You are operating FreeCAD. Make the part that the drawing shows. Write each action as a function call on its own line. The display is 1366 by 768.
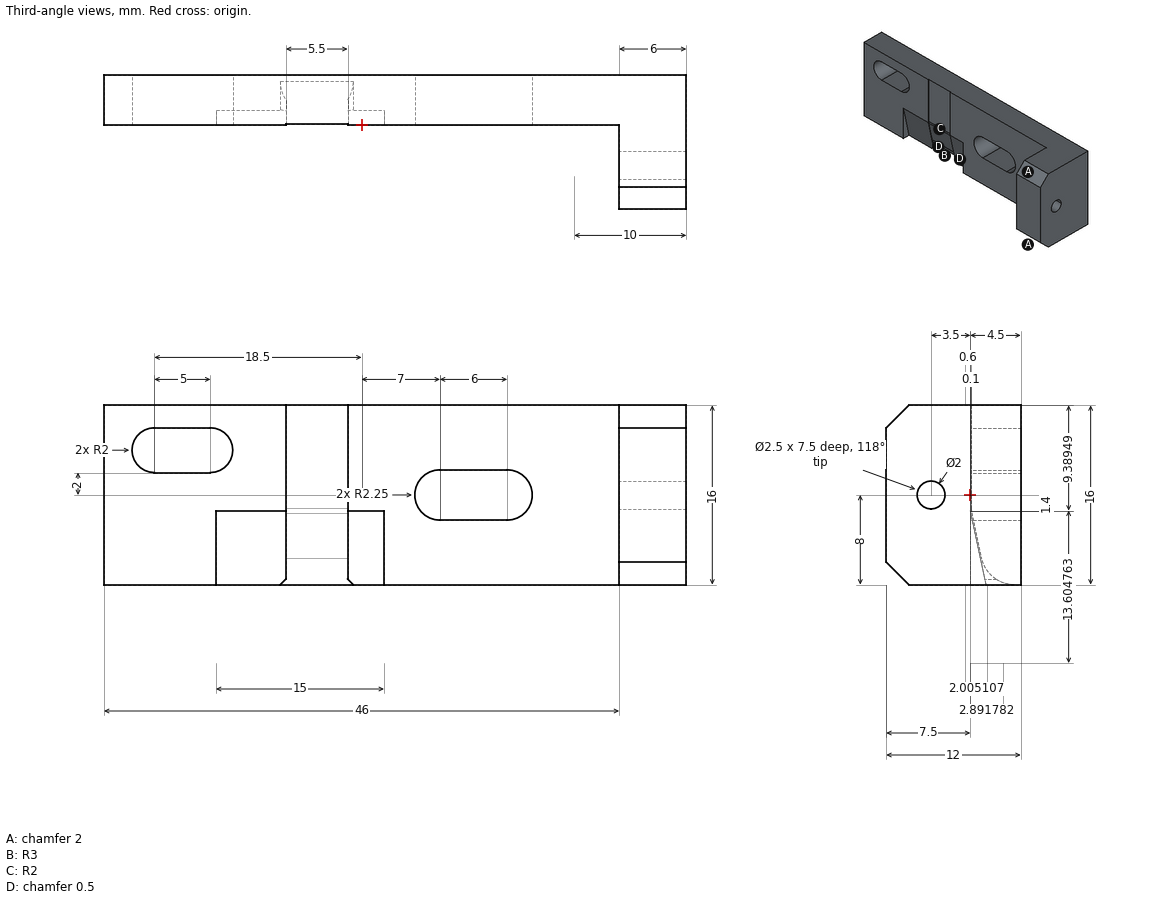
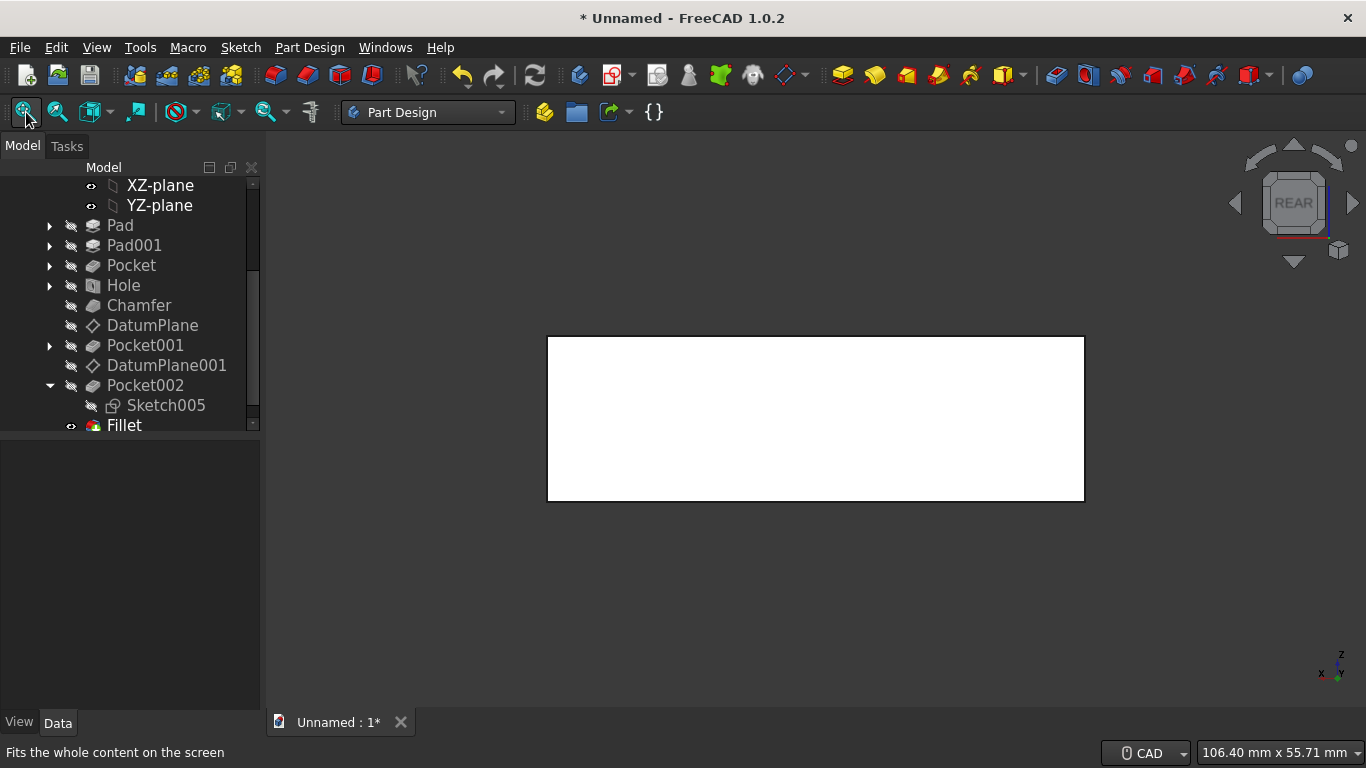
key(6)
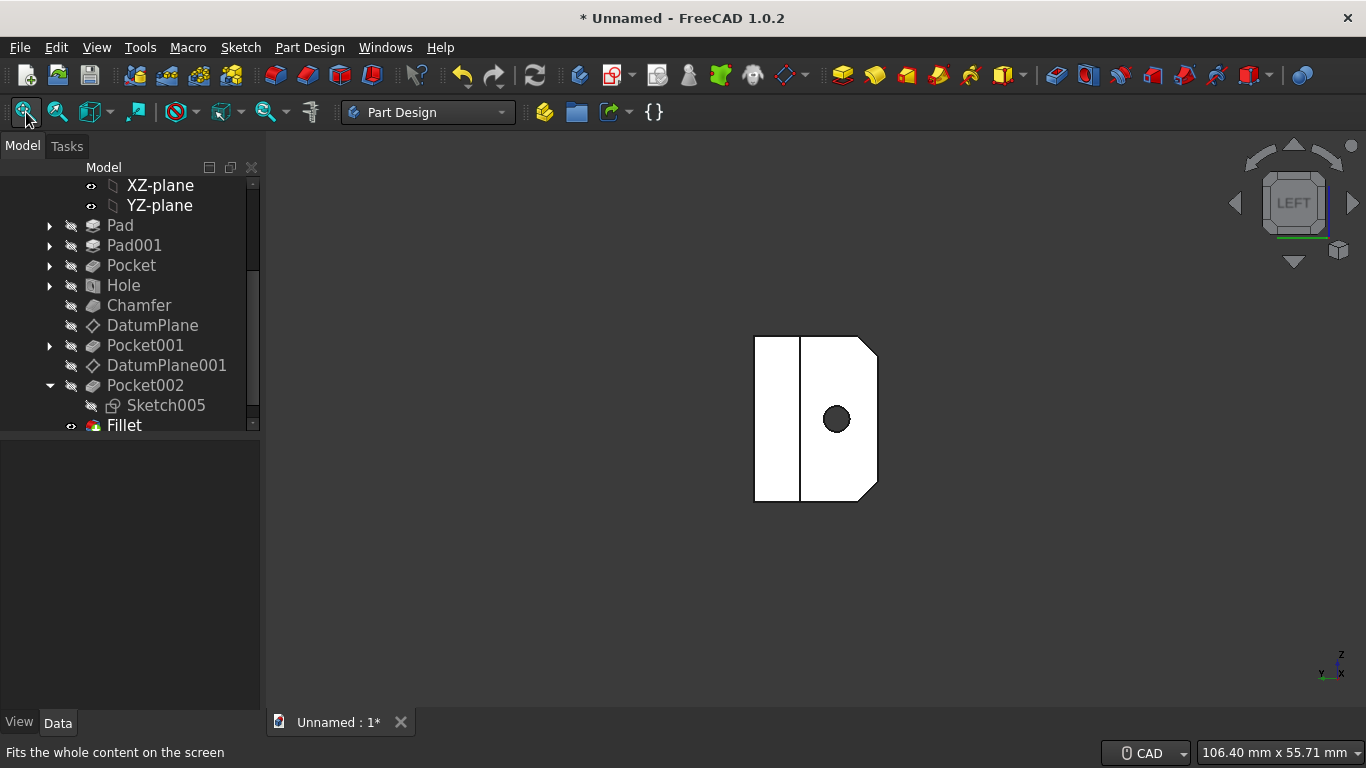
key(v)
key(f)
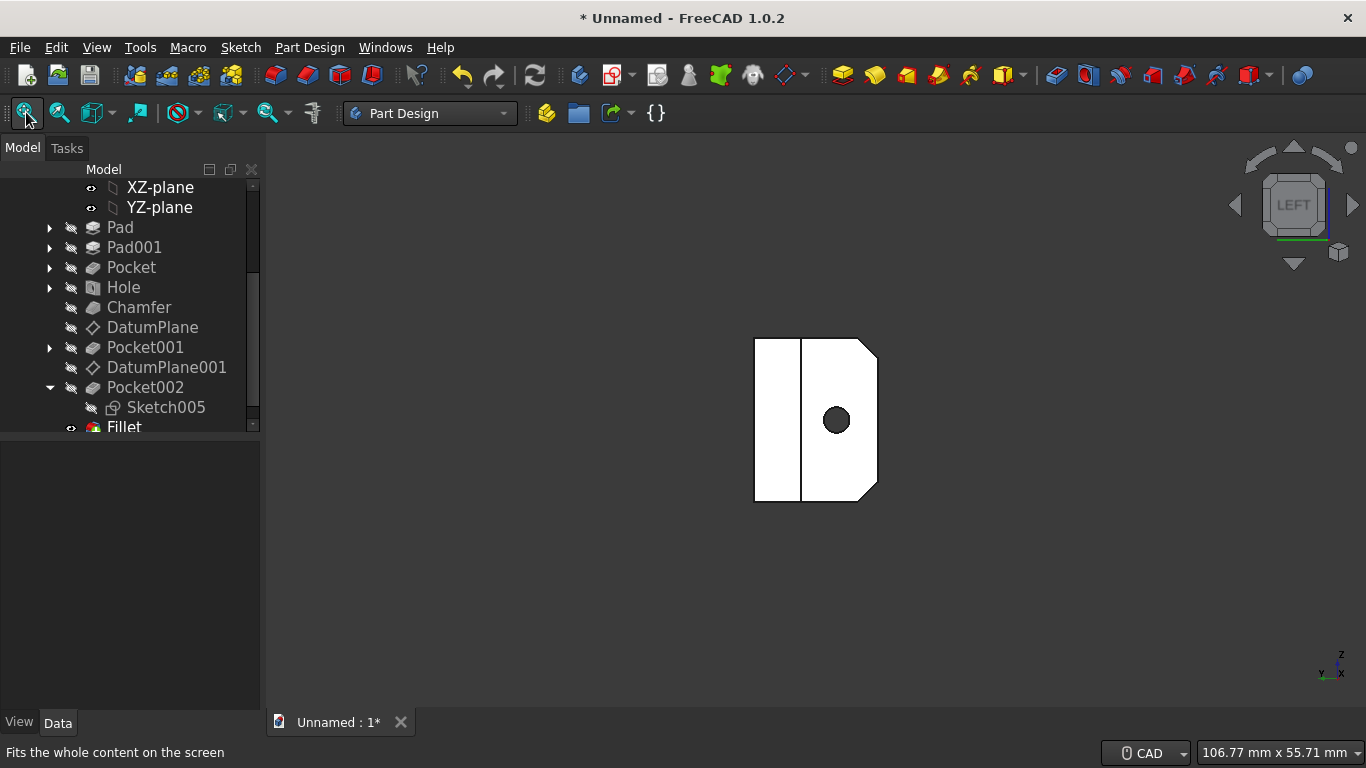
key(v)
key(3)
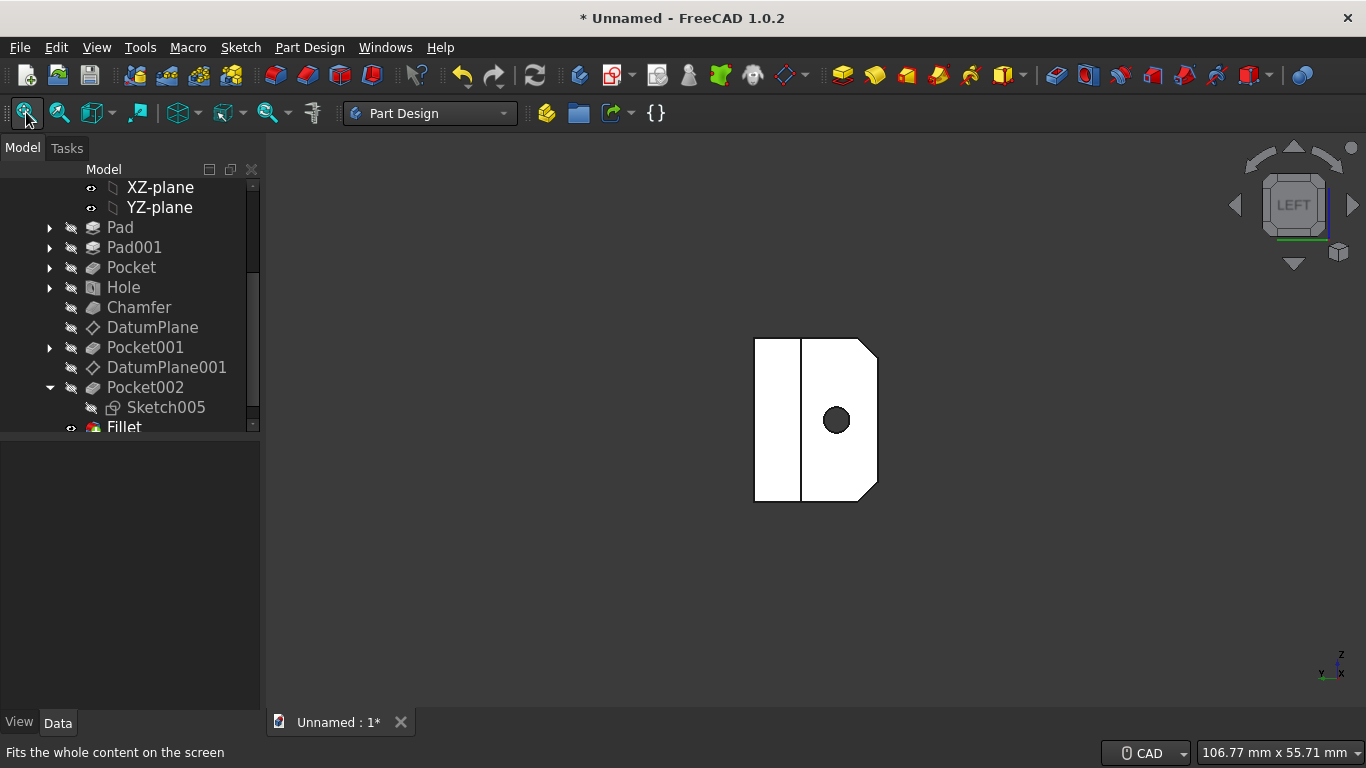
key(0)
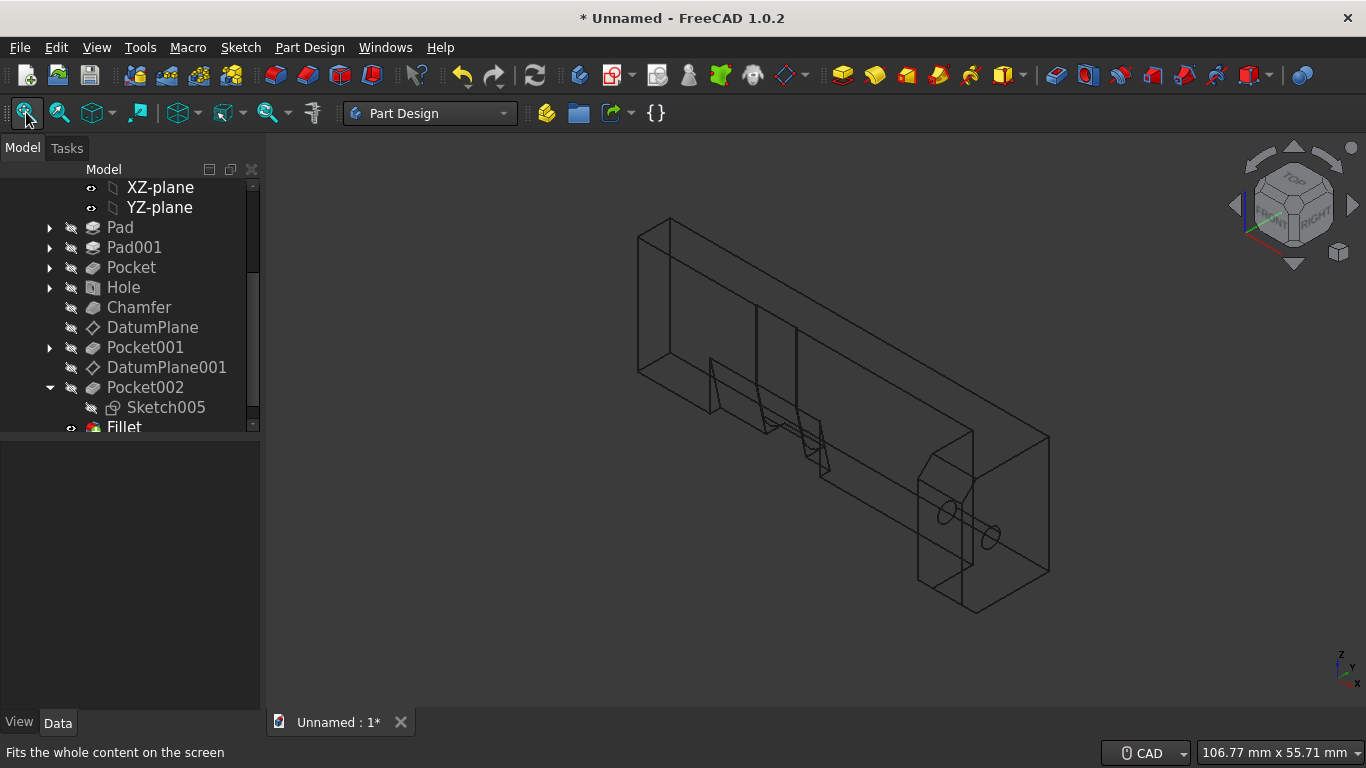
click(777, 395)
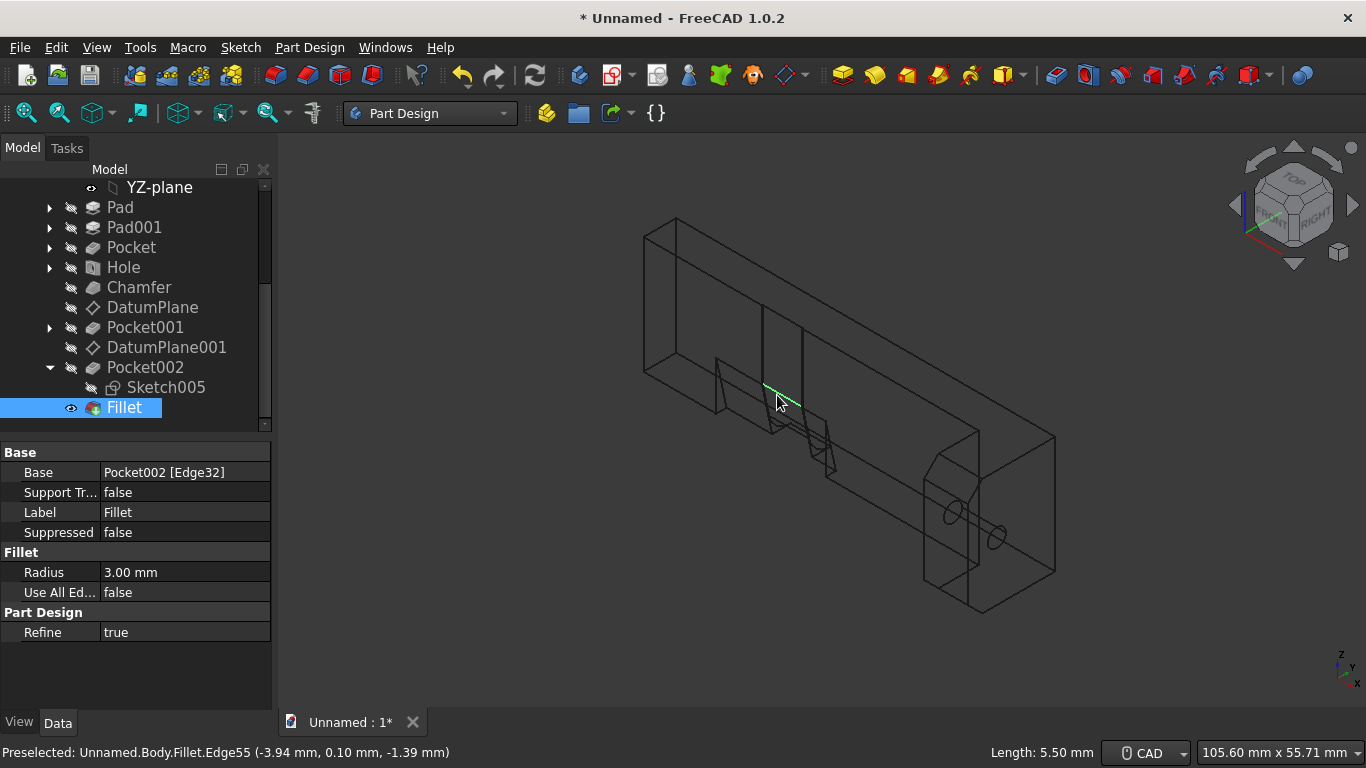
key(v)
key(1)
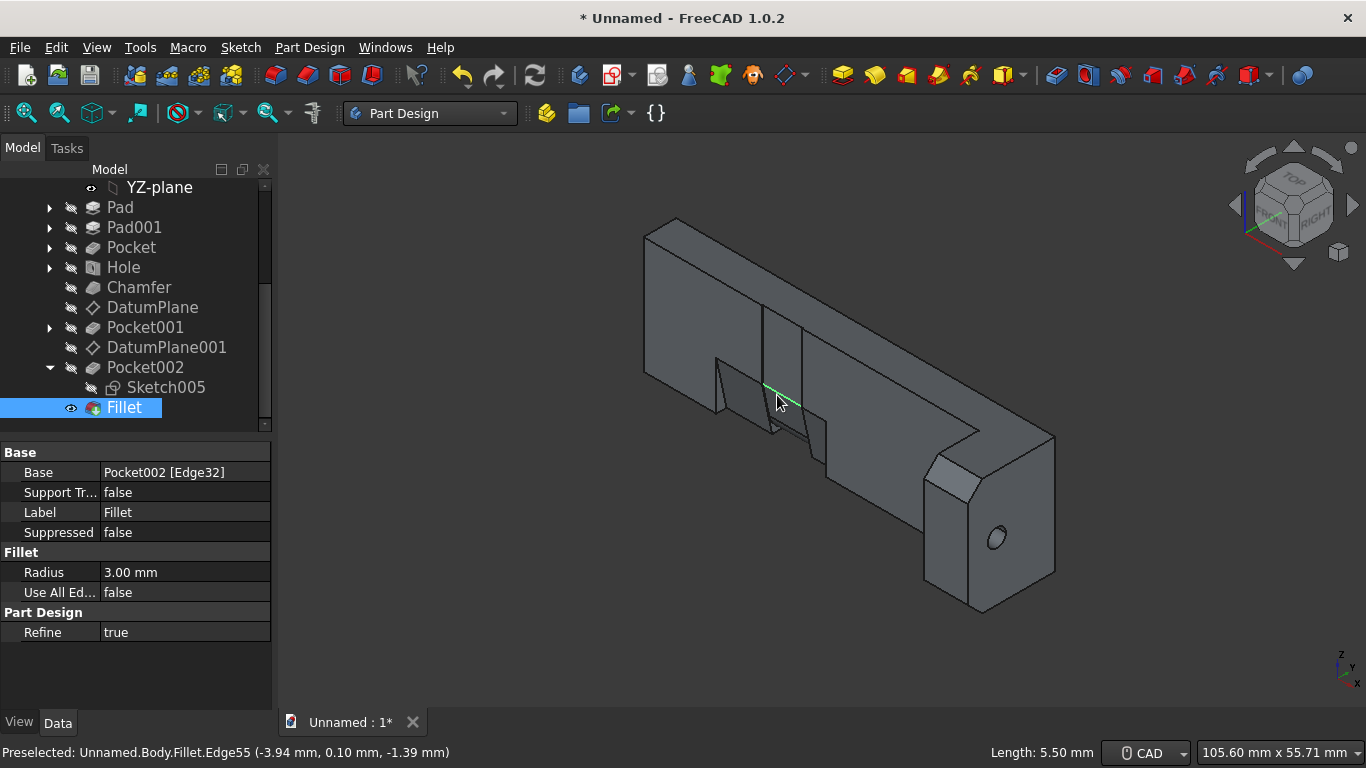
click(276, 76)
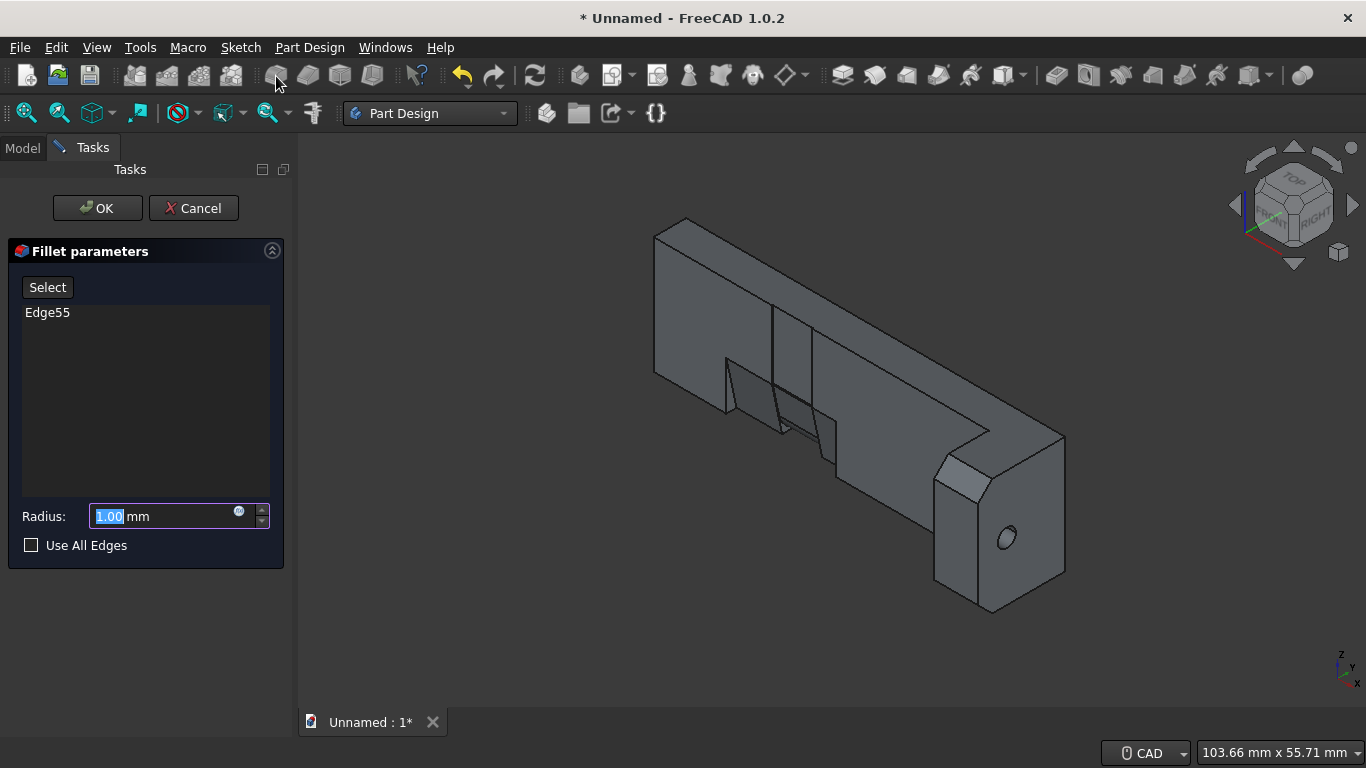
text(2)
key(Tab)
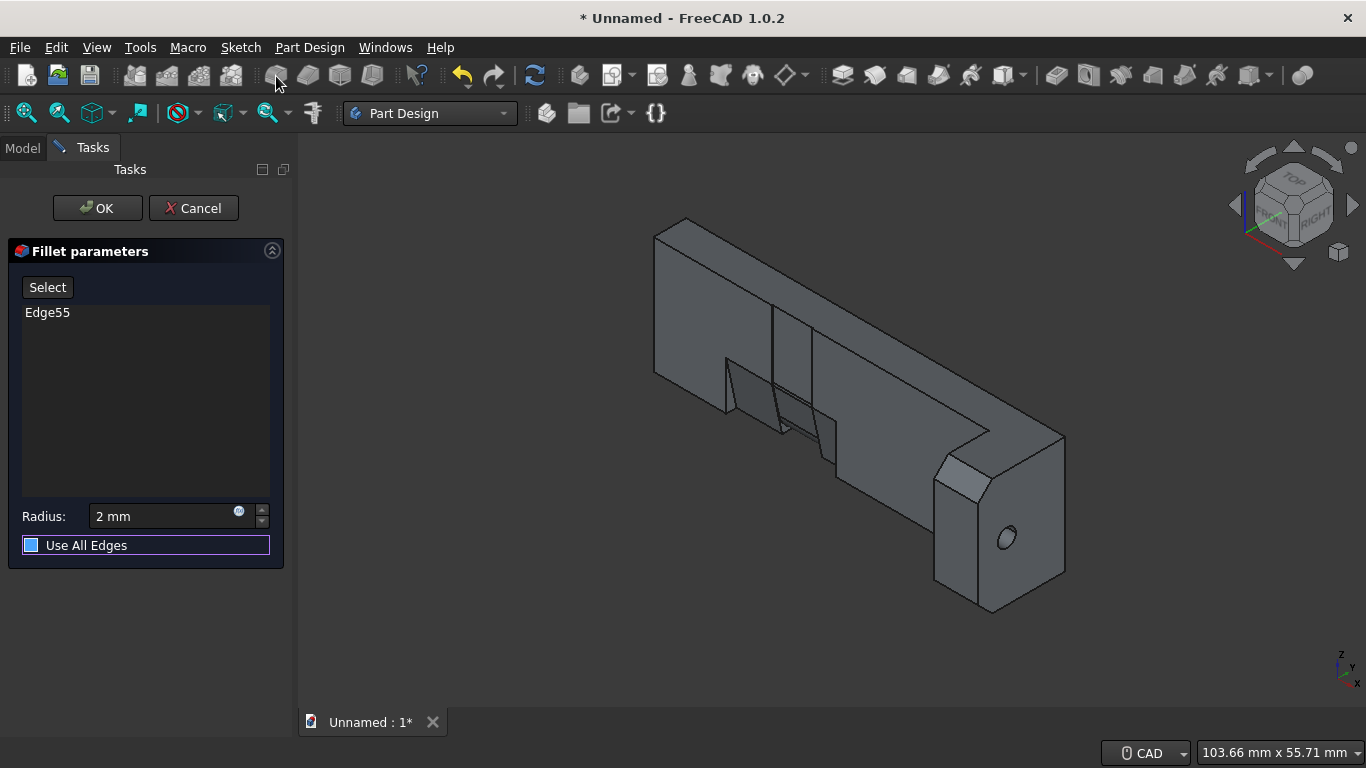
click(98, 208)